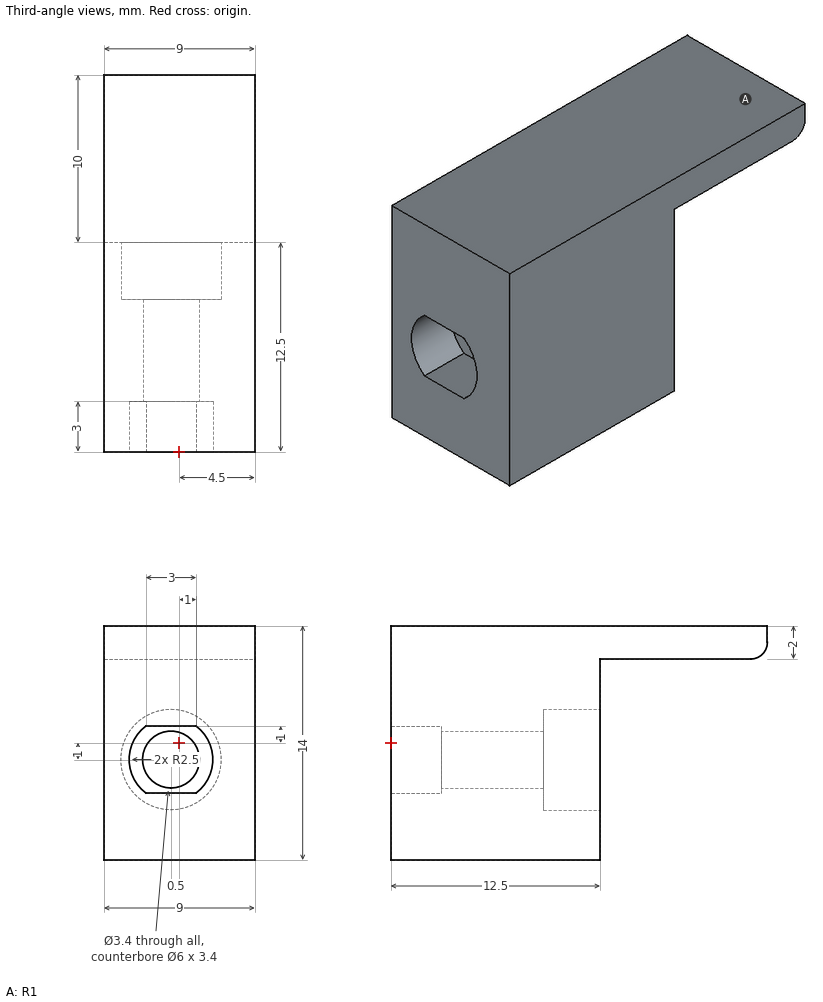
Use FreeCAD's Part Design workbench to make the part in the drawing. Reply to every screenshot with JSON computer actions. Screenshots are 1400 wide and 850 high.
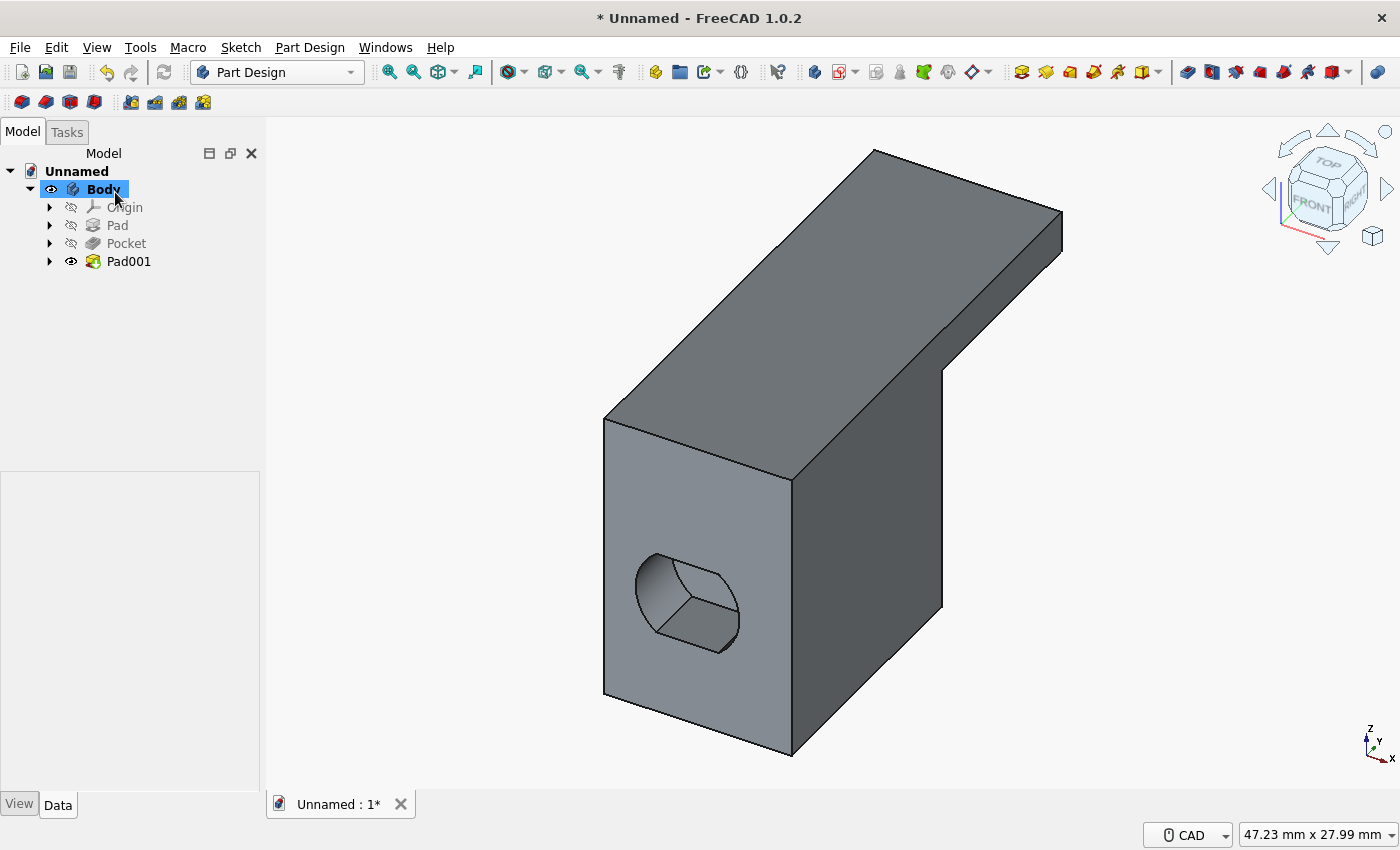
{"action": "key", "text": "0"}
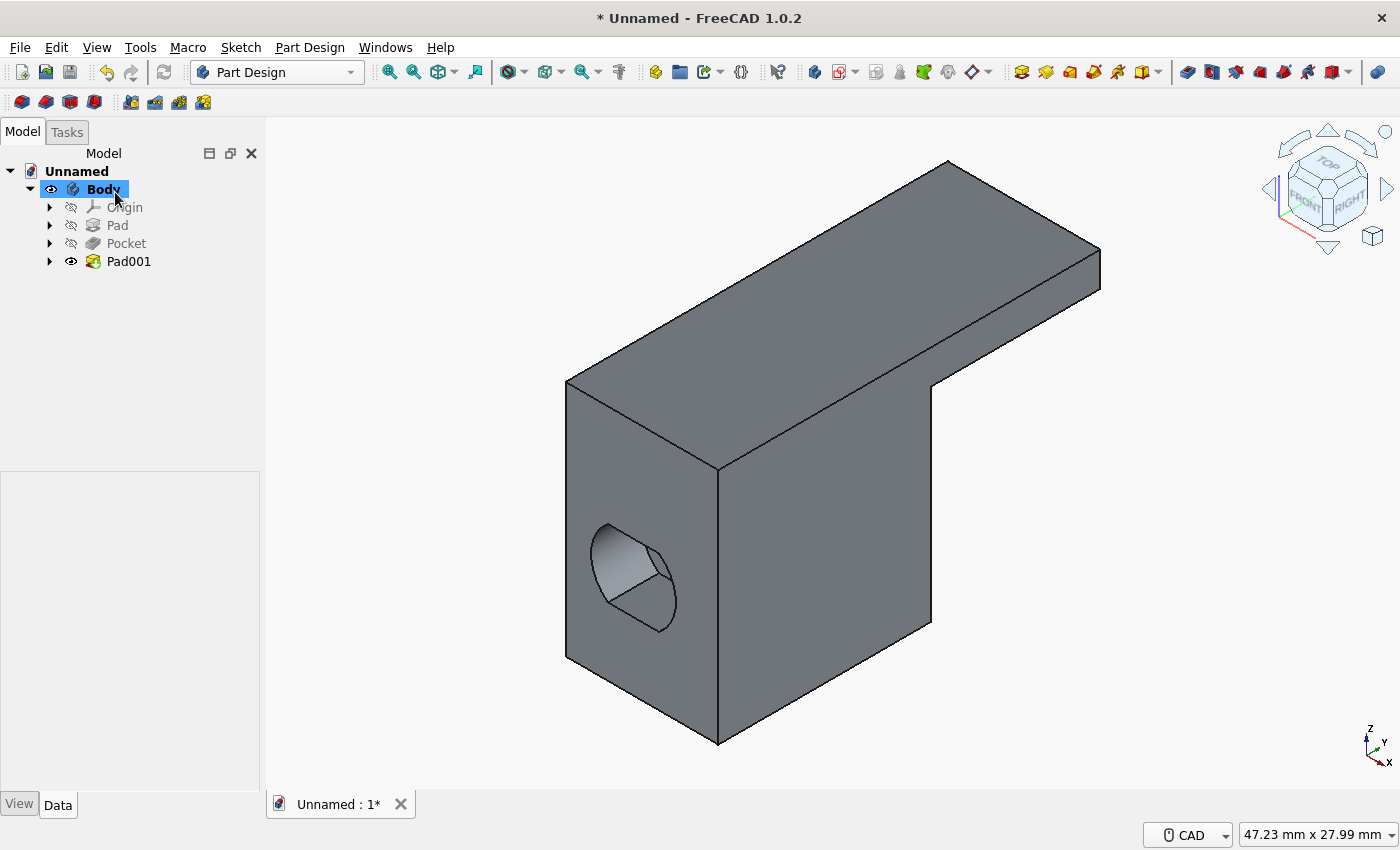
{"action": "key", "text": "2"}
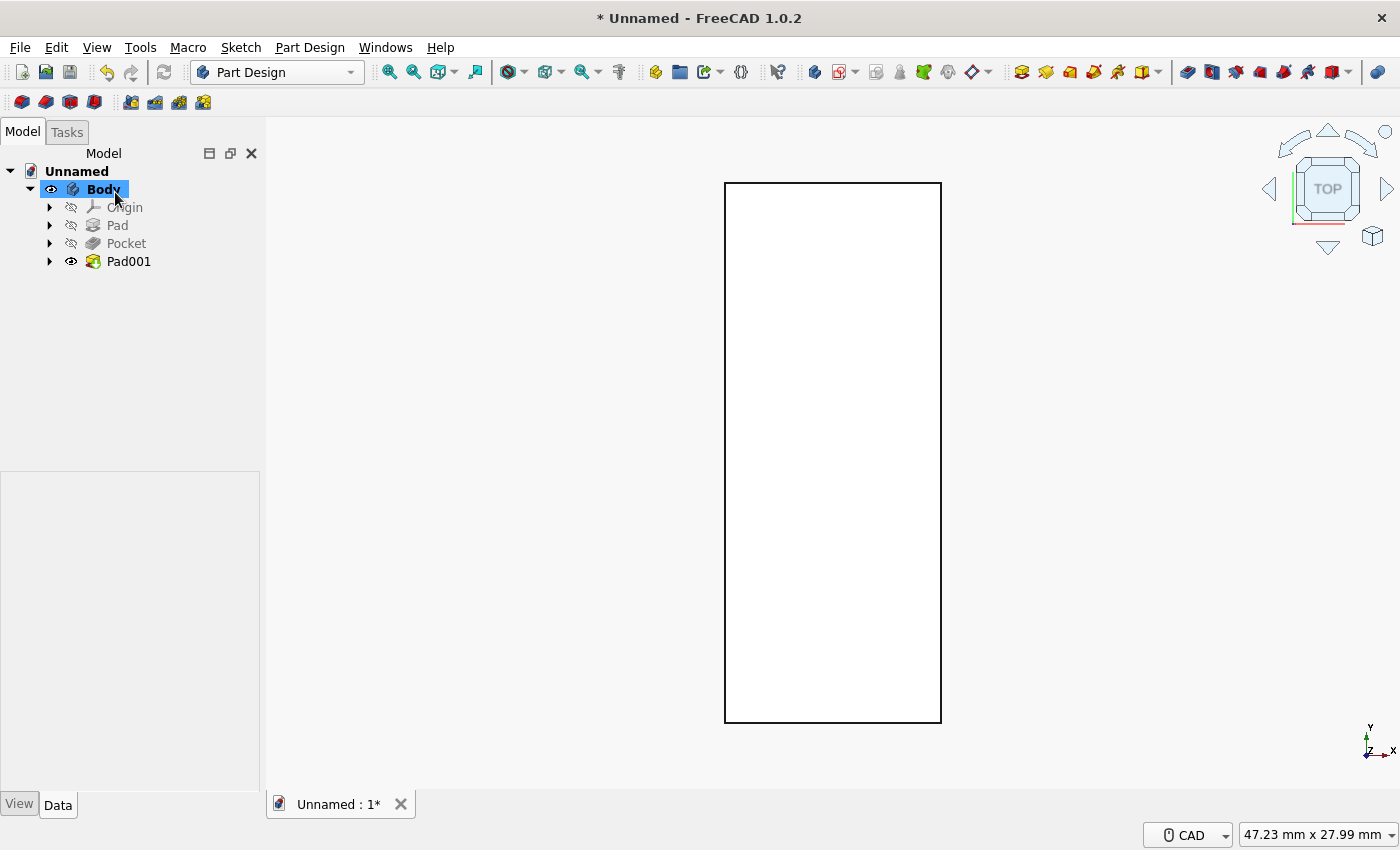
{"action": "key", "text": "1"}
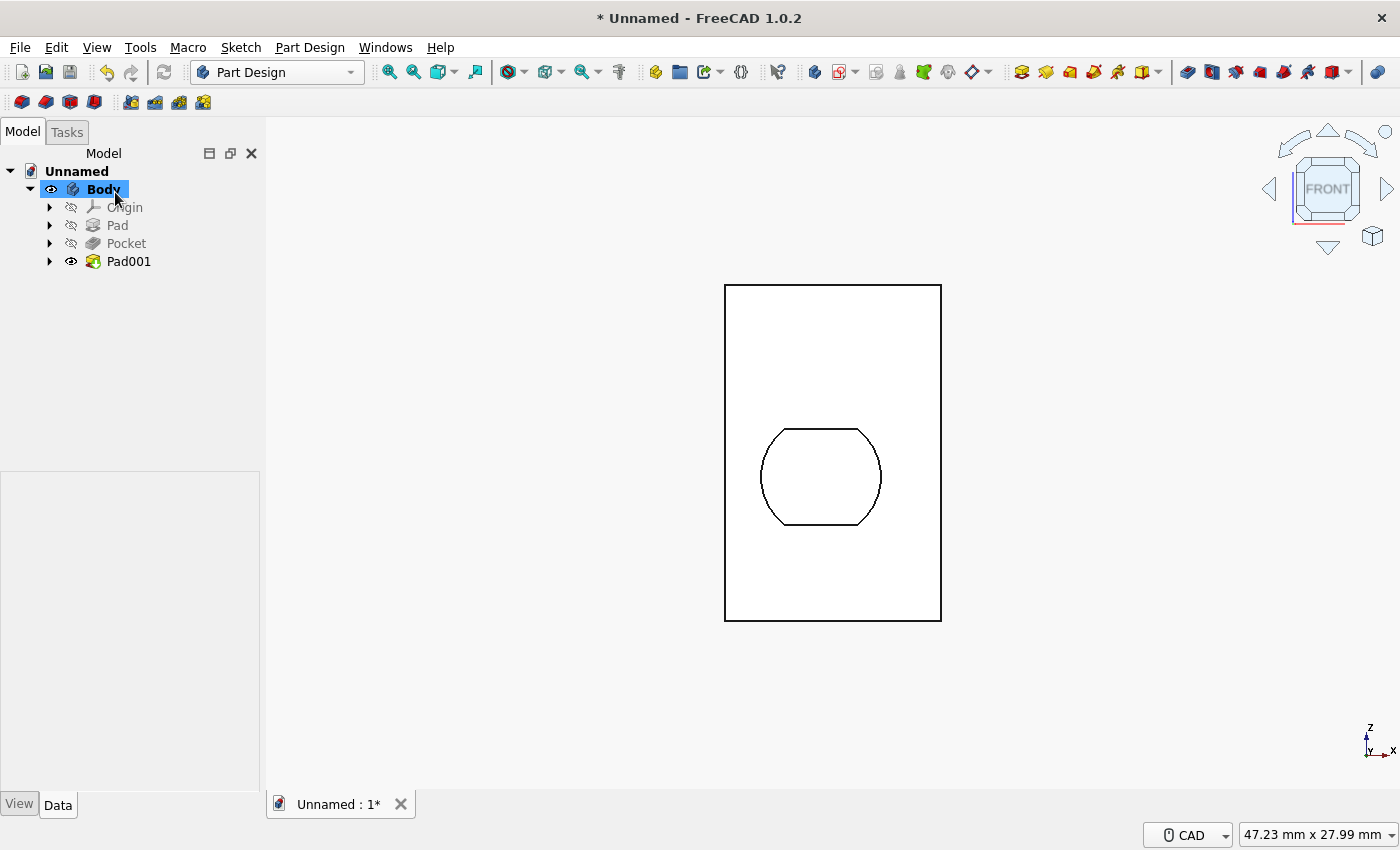
{"action": "key", "text": "3"}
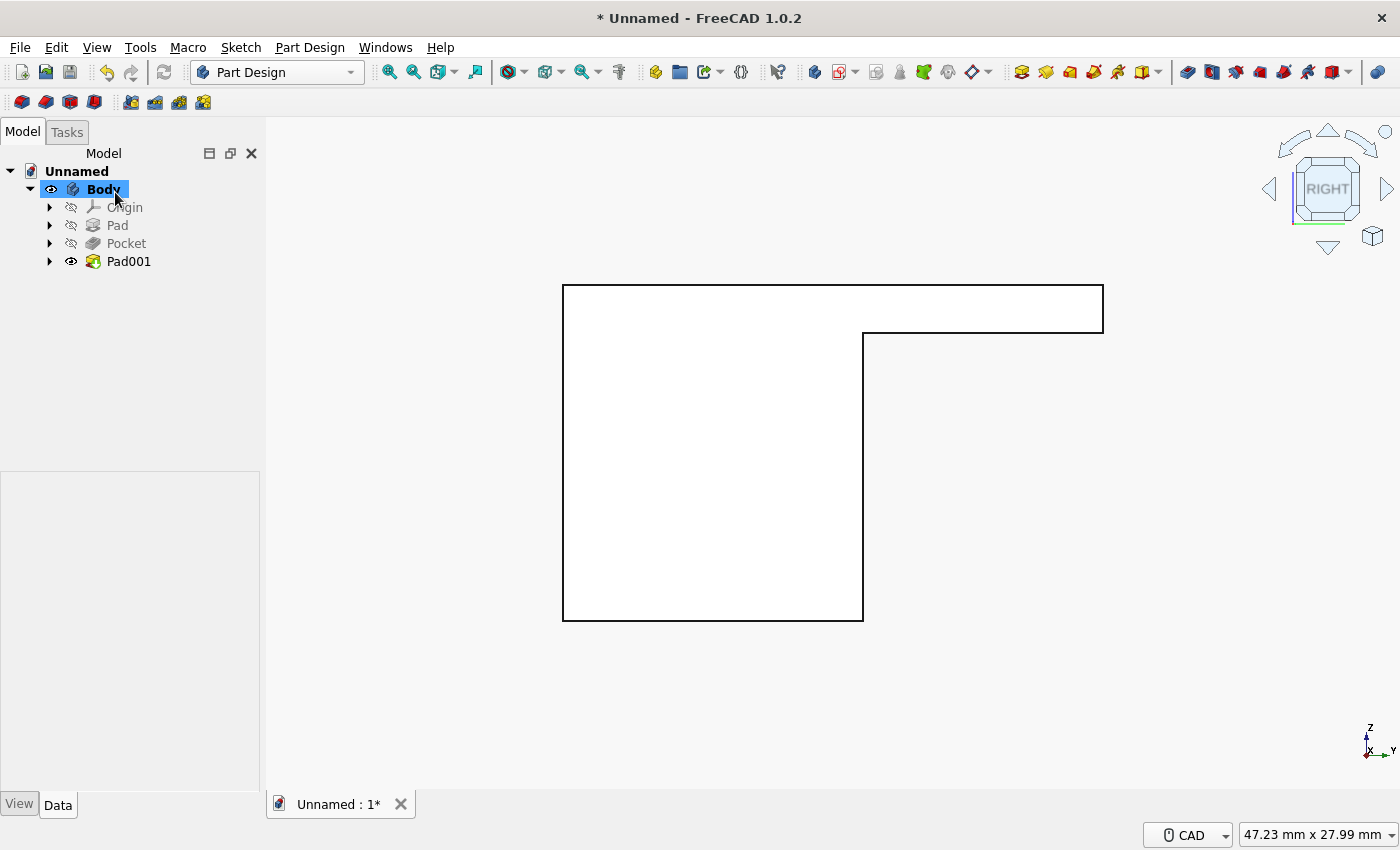
{"action": "key", "text": "5"}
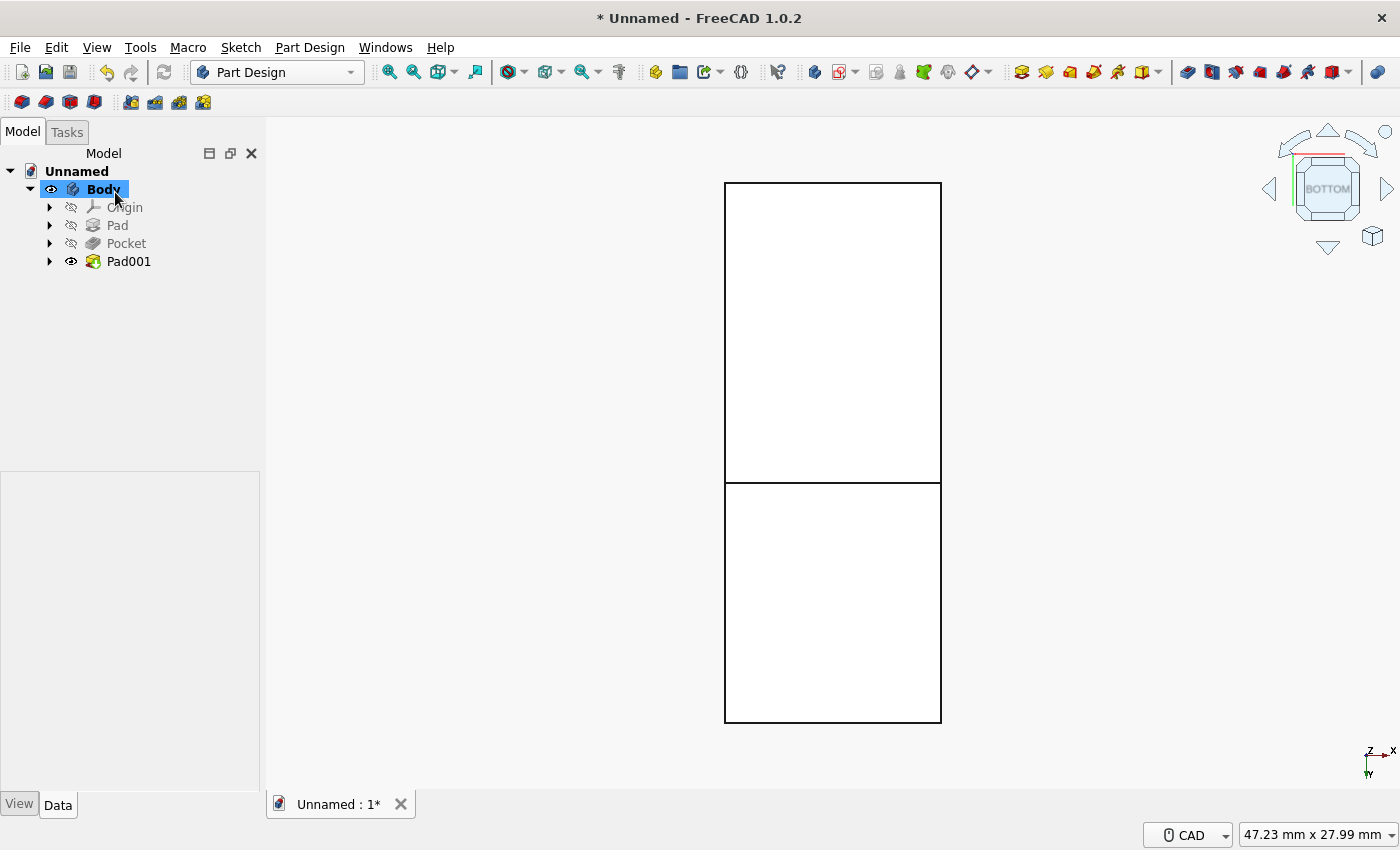
{"action": "key", "text": "4"}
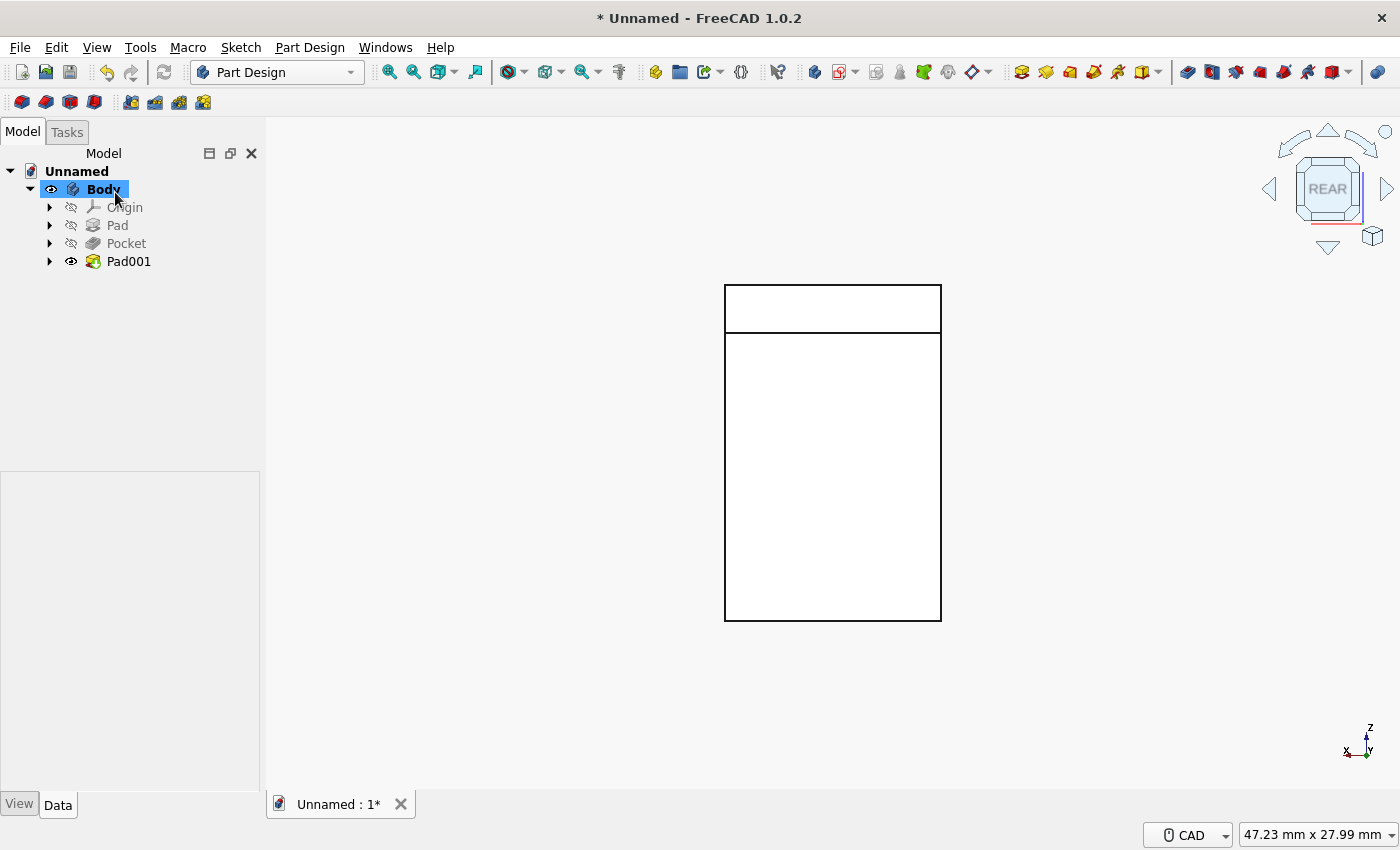
{"action": "left_click", "coordinate": [833, 332]}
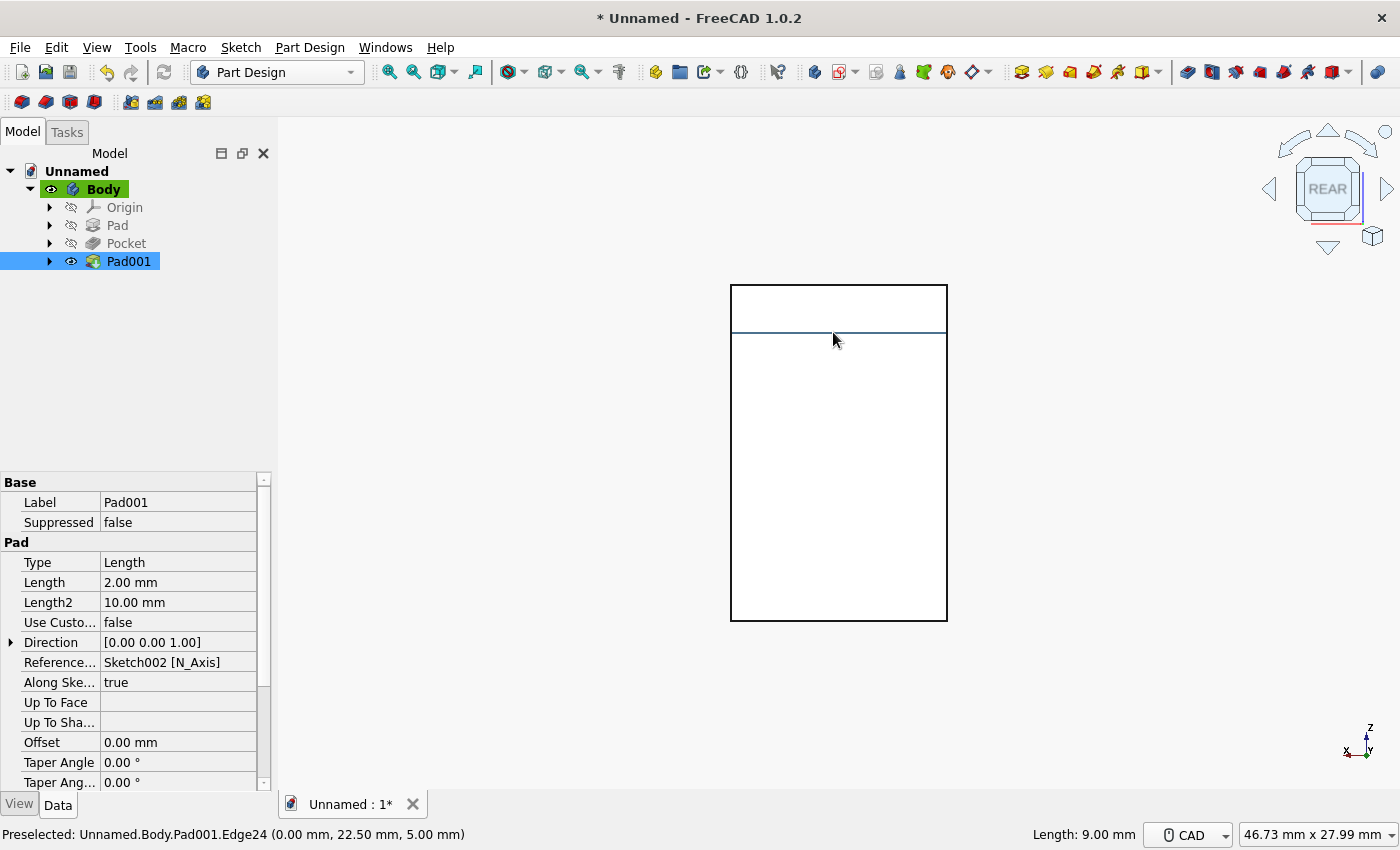
{"action": "left_click", "coordinate": [22, 102]}